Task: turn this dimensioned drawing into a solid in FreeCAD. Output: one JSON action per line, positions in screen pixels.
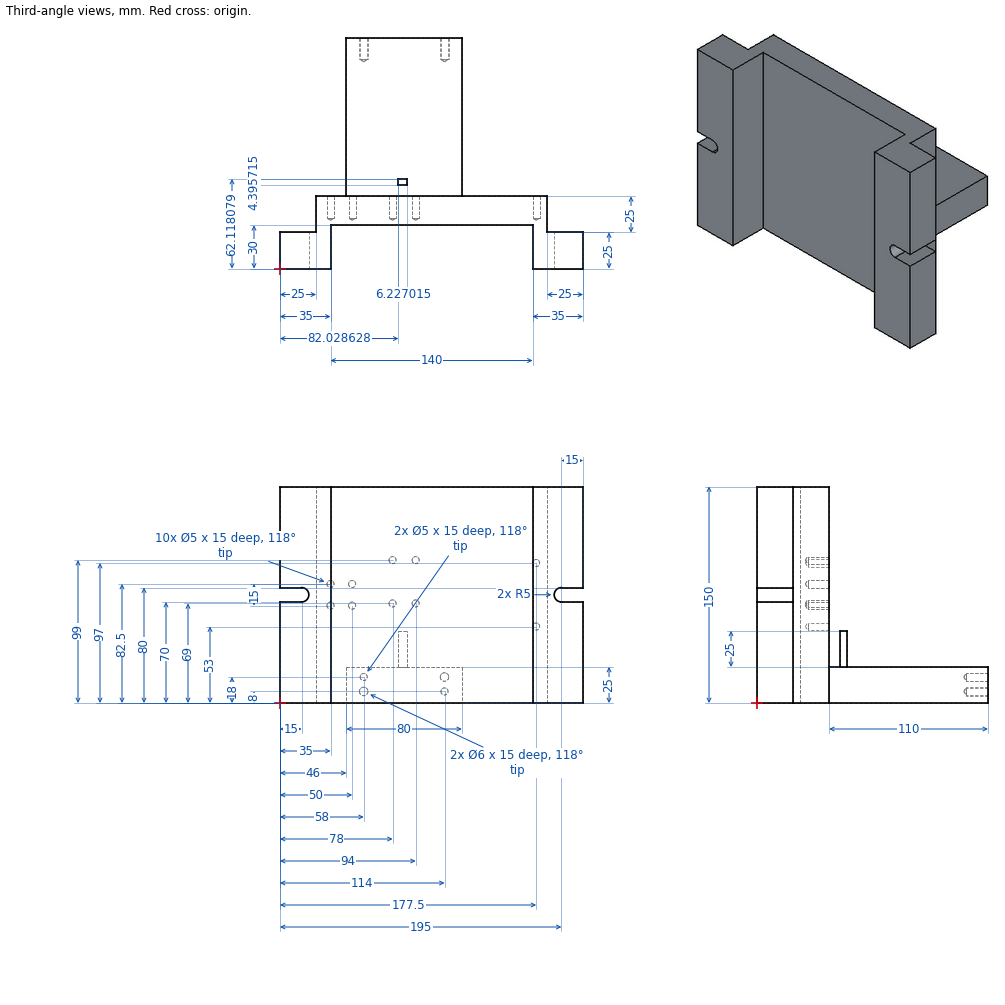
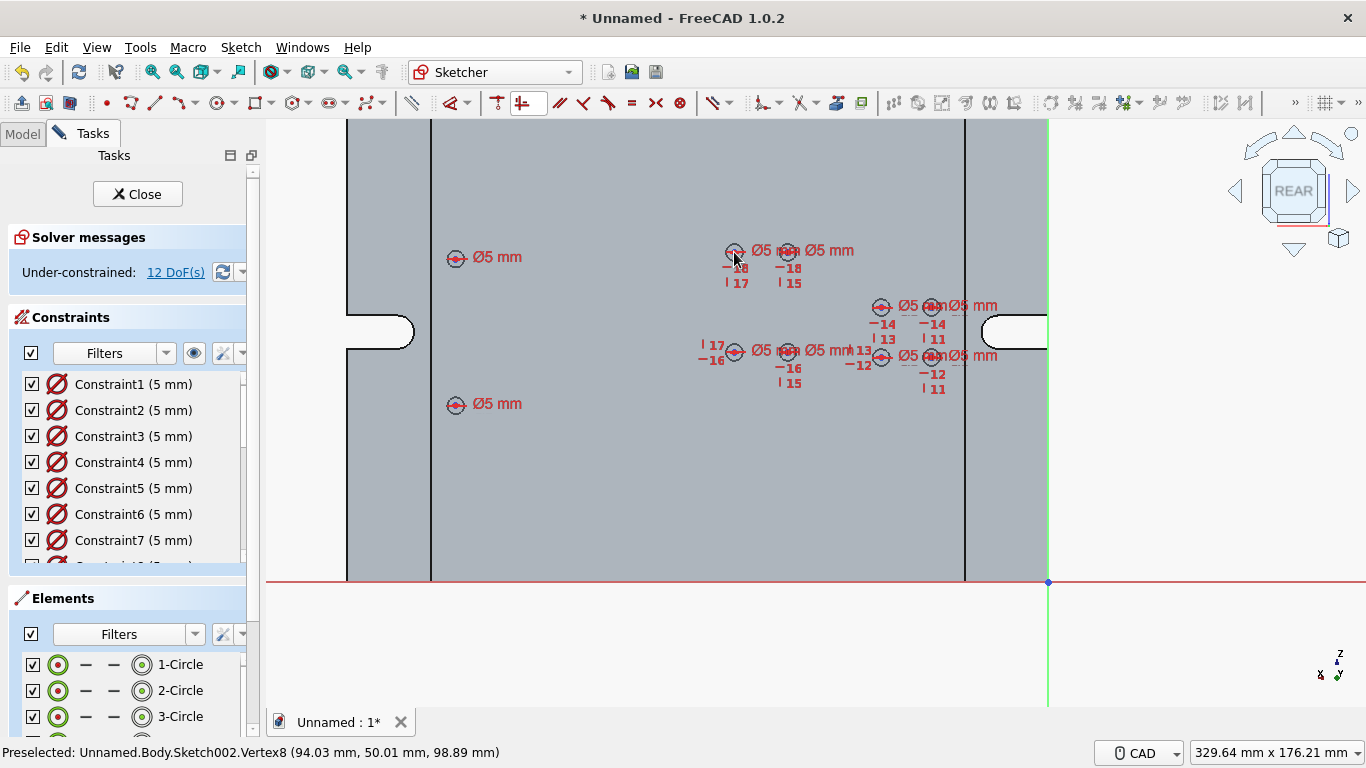
{"action": "left_click", "coordinate": [456, 259]}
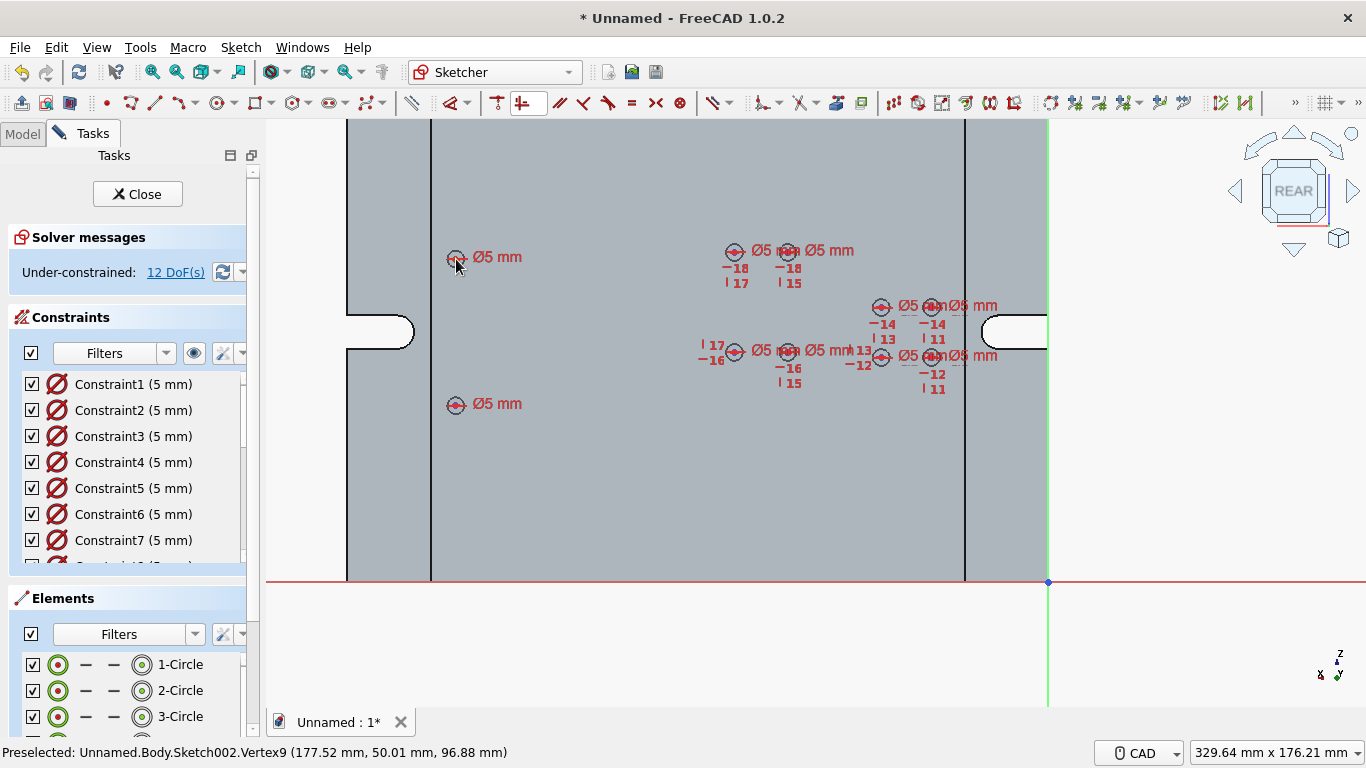
{"action": "left_click", "coordinate": [456, 406]}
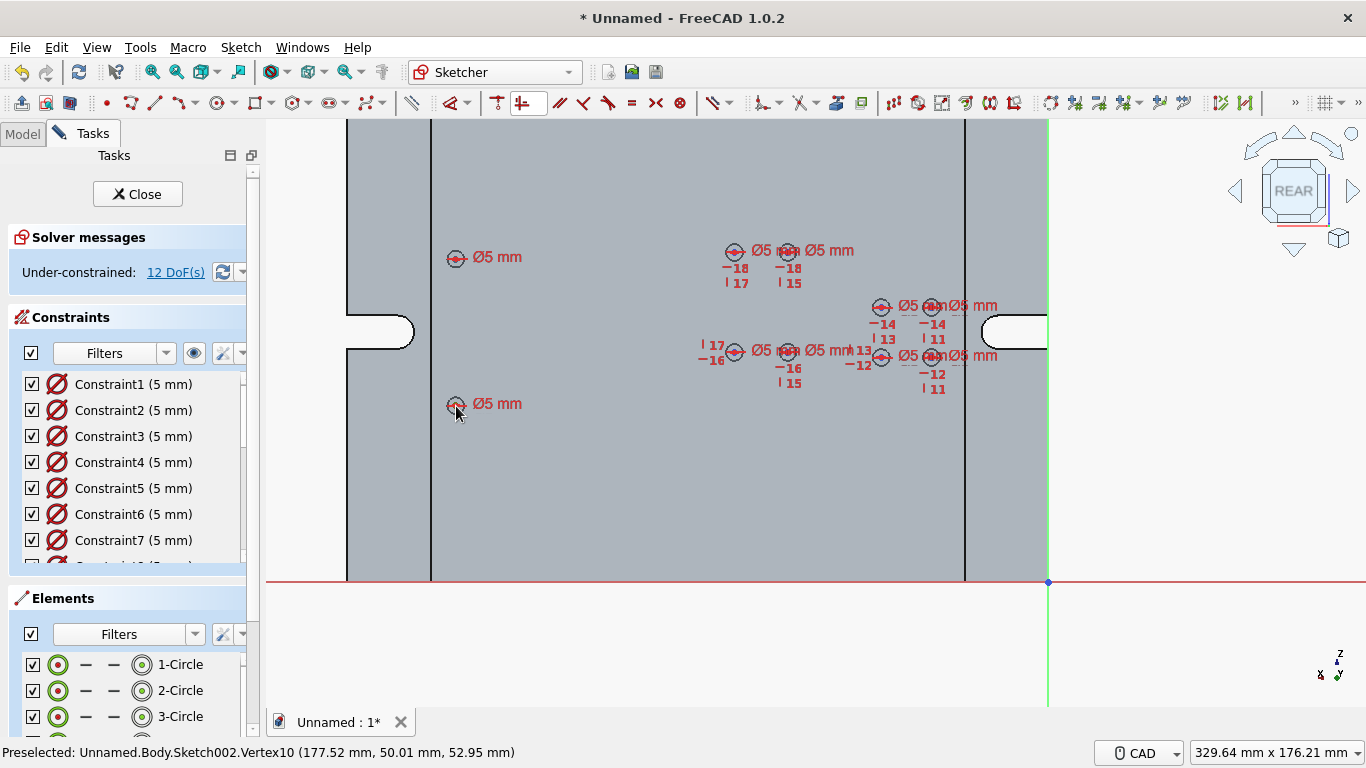
{"action": "key", "text": "v"}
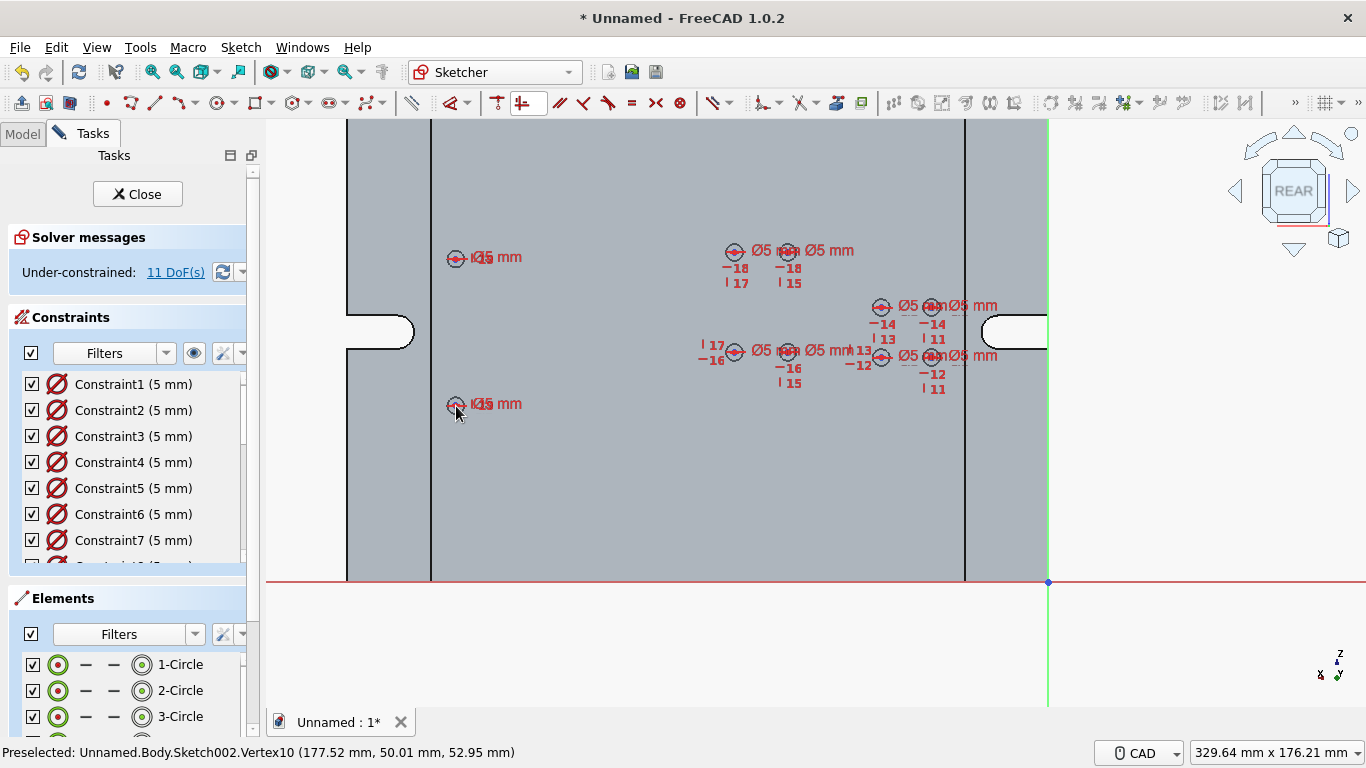
{"action": "key", "text": "d"}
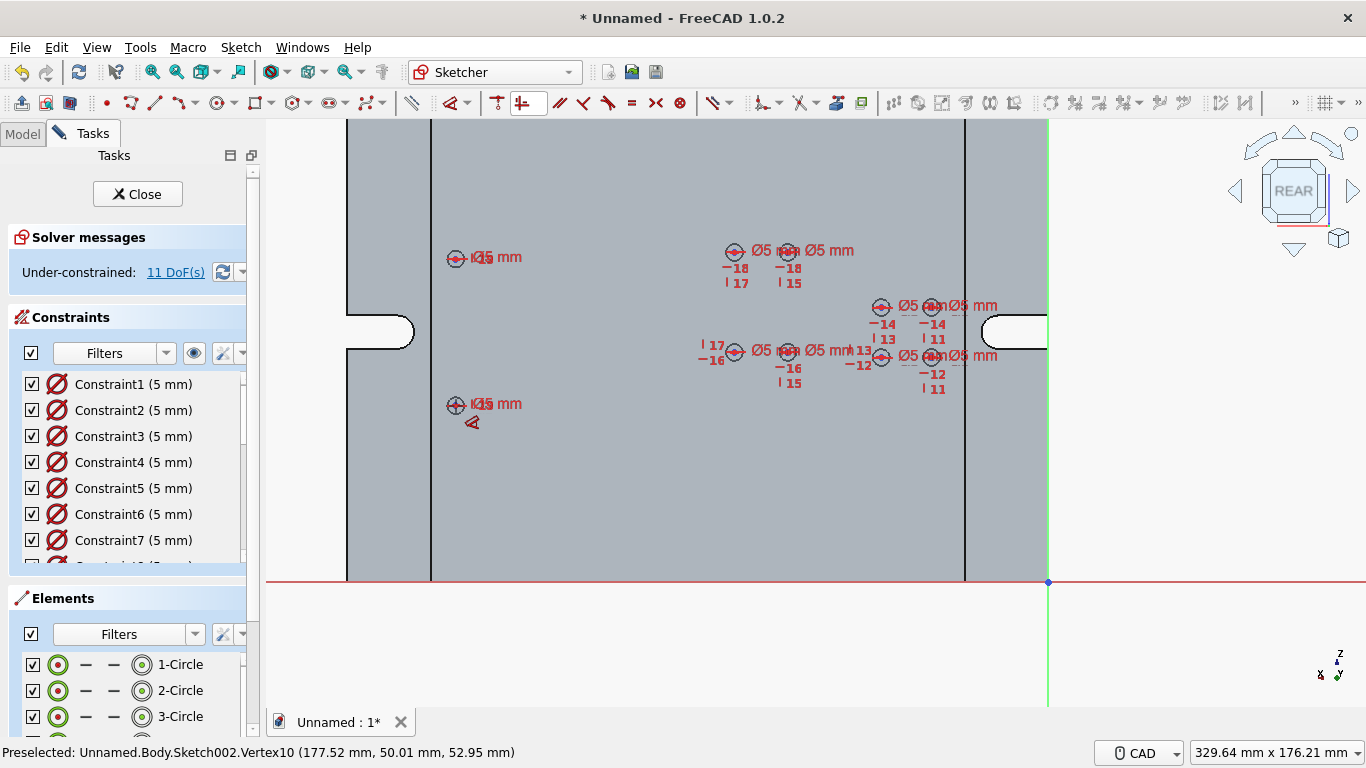
{"action": "left_click", "coordinate": [932, 308]}
{"action": "left_click", "coordinate": [990, 616]}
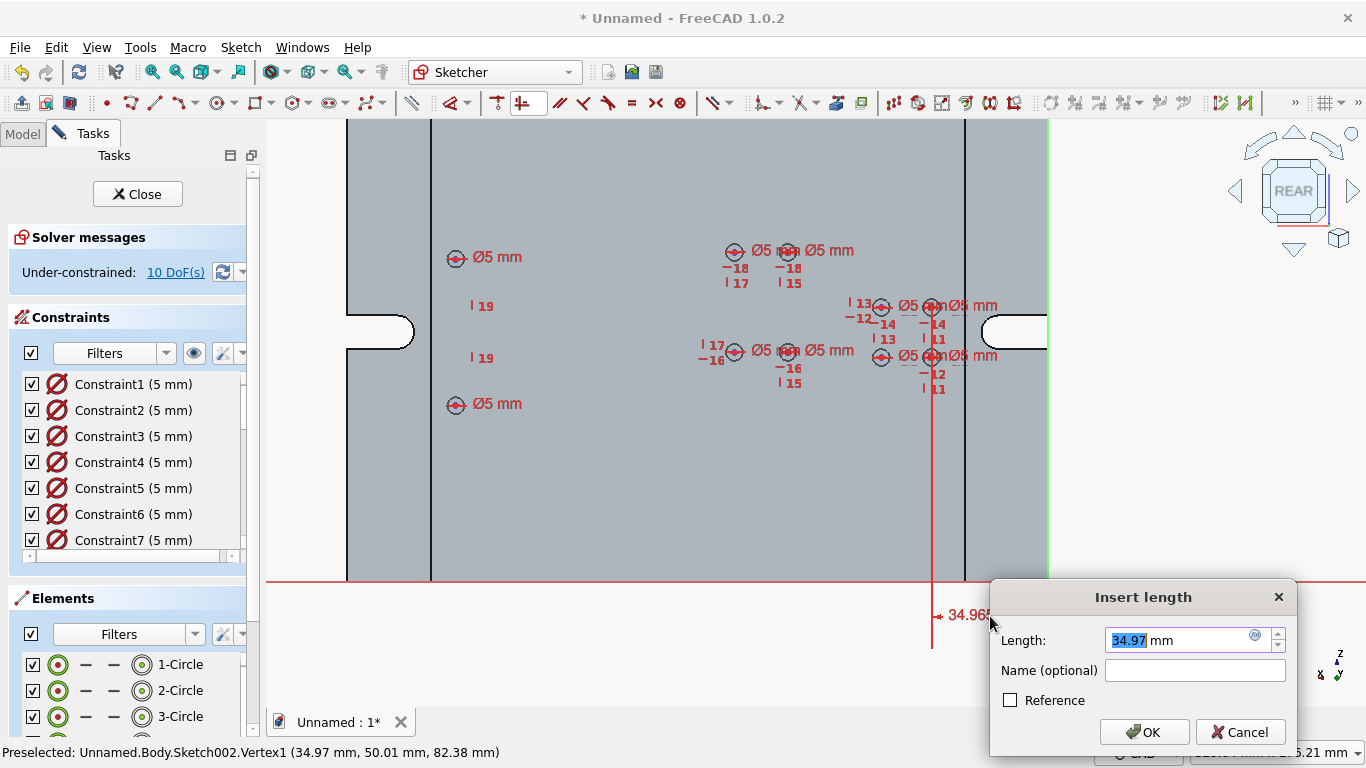
{"action": "type", "text": "35"}
{"action": "key", "text": "Return"}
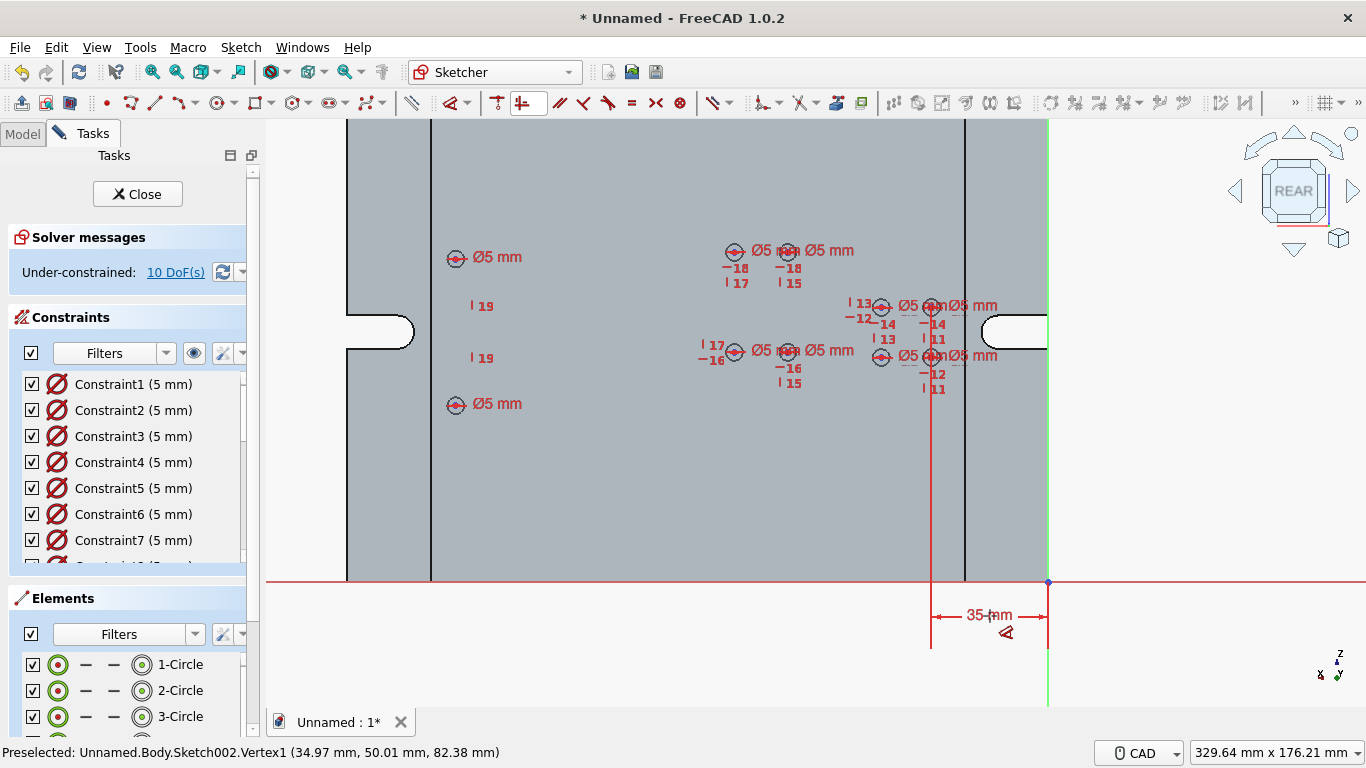
{"action": "left_click", "coordinate": [881, 358]}
{"action": "left_click", "coordinate": [906, 616]}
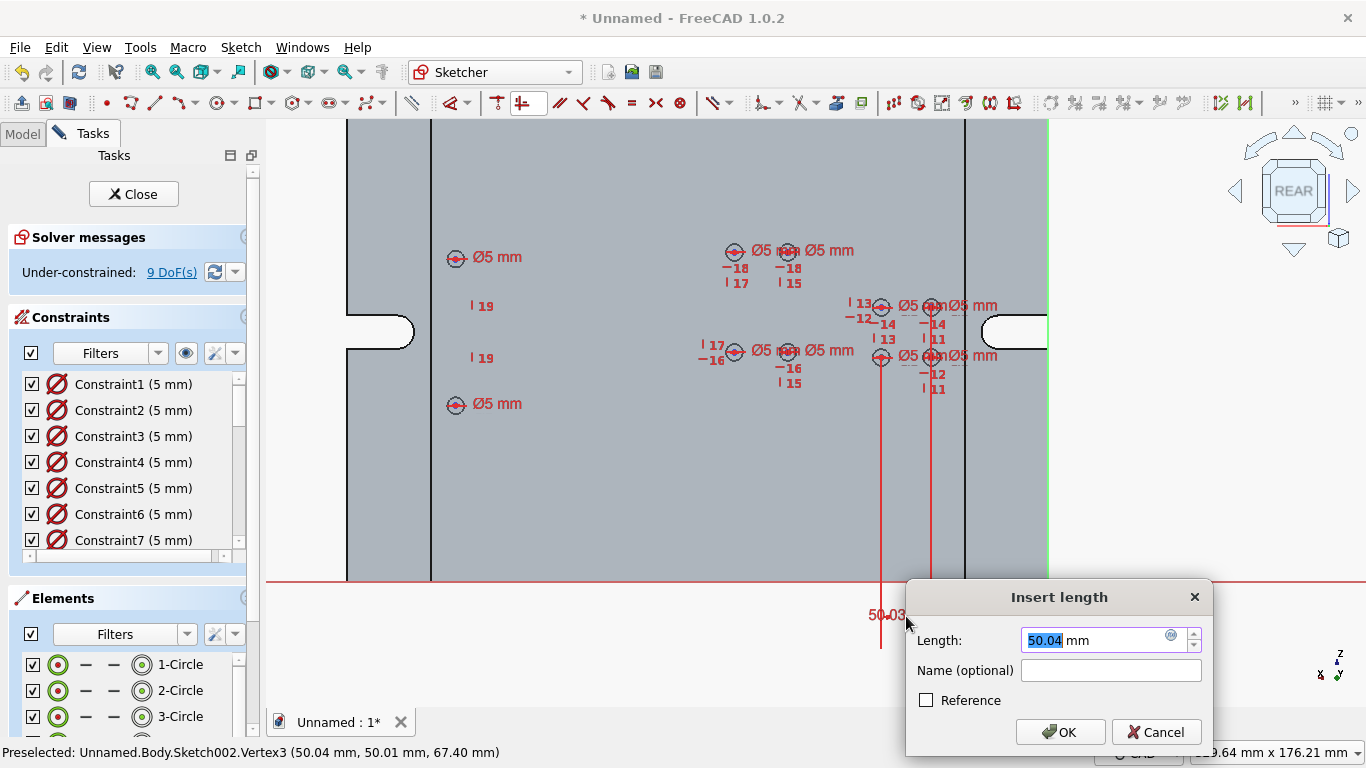
{"action": "type", "text": "50"}
{"action": "key", "text": "Return"}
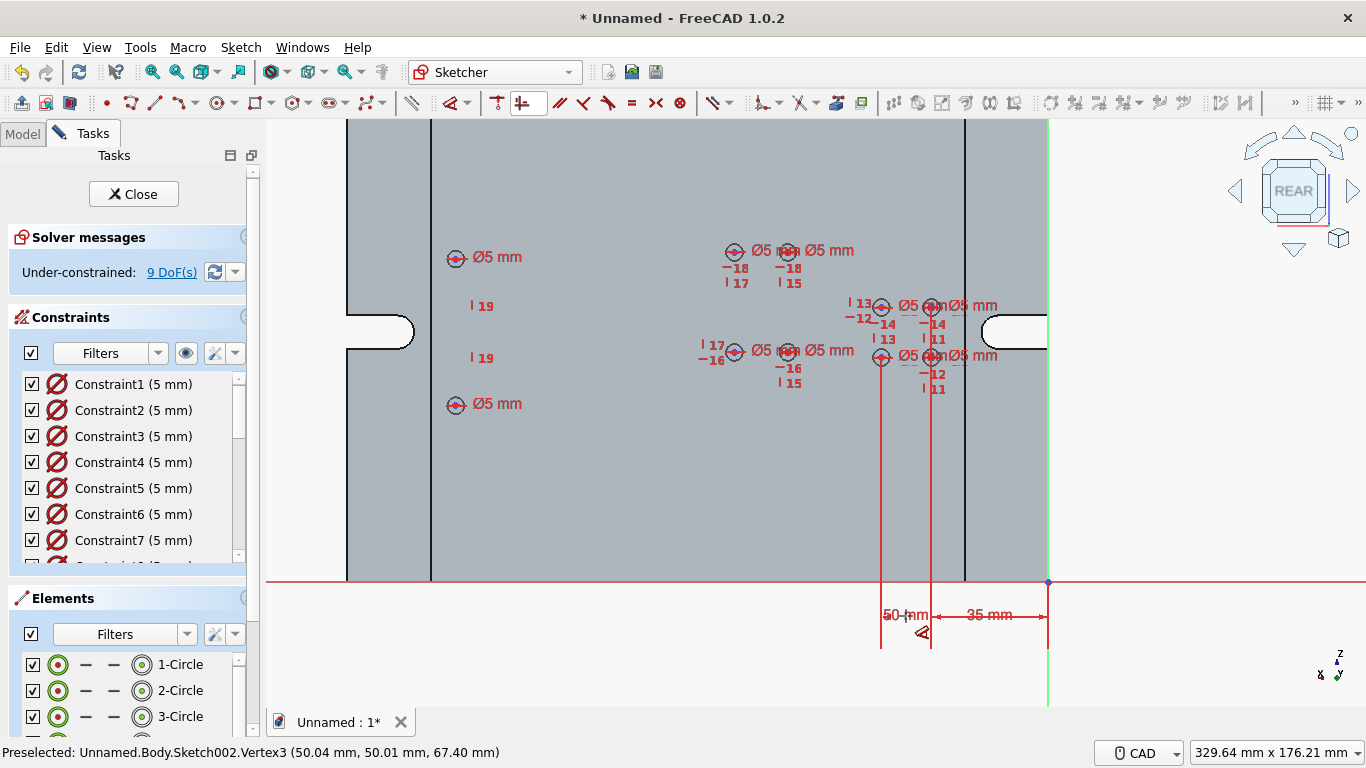
{"action": "left_click", "coordinate": [788, 352]}
{"action": "left_click", "coordinate": [827, 616]}